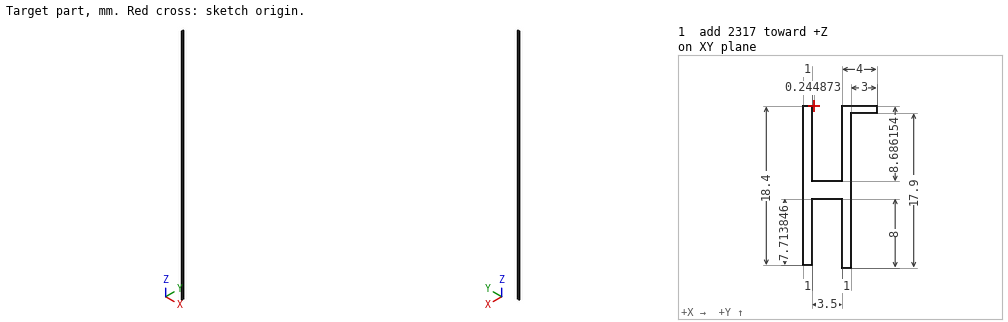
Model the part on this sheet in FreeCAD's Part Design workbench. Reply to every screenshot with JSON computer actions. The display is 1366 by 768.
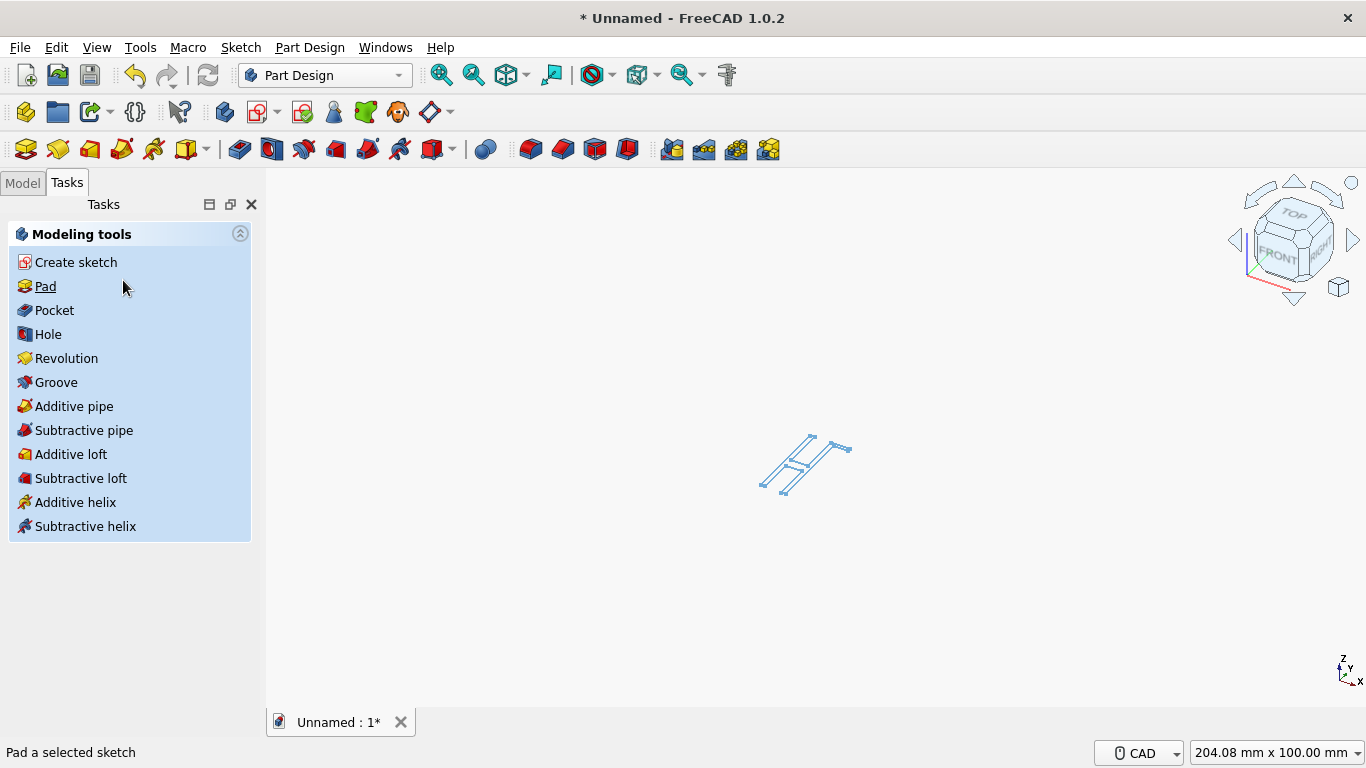
{"action": "left_click", "coordinate": [26, 150]}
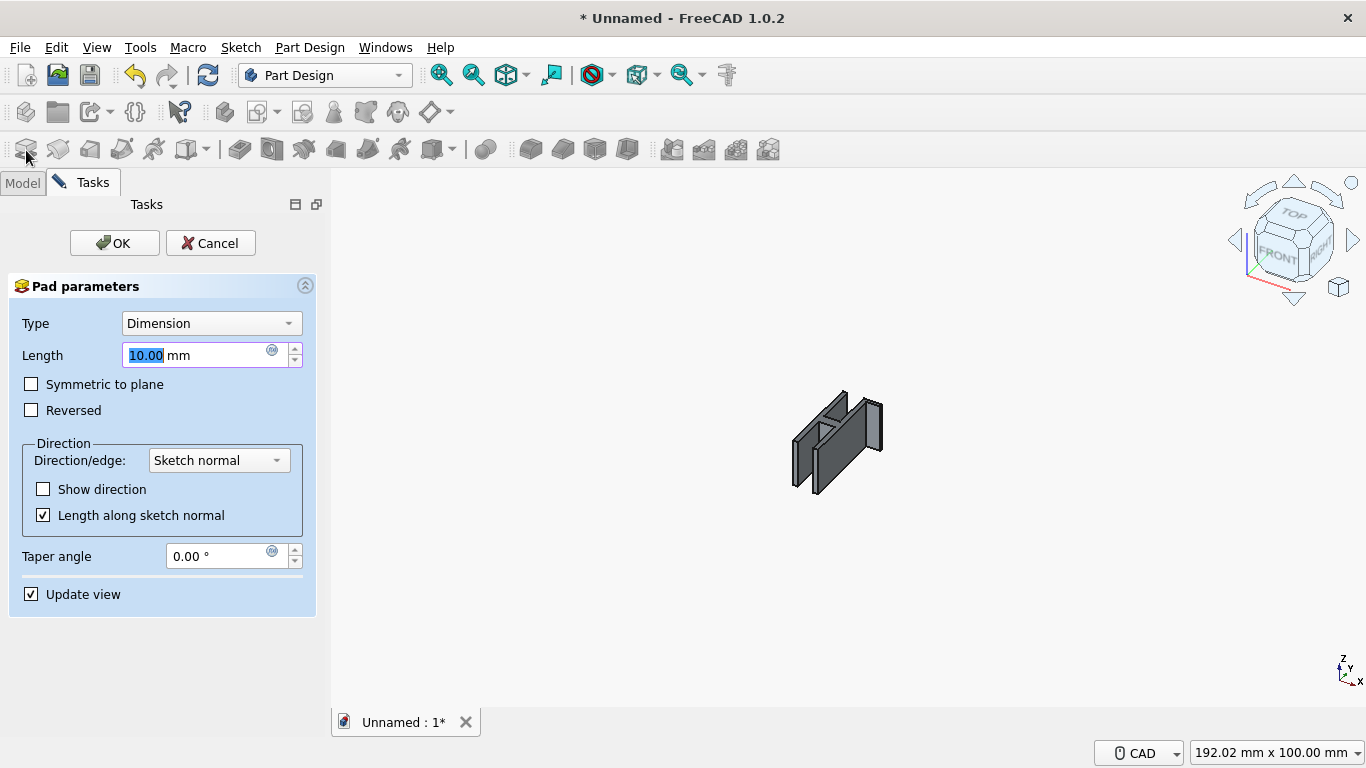
{"action": "type", "text": "2317"}
{"action": "key", "text": "Tab"}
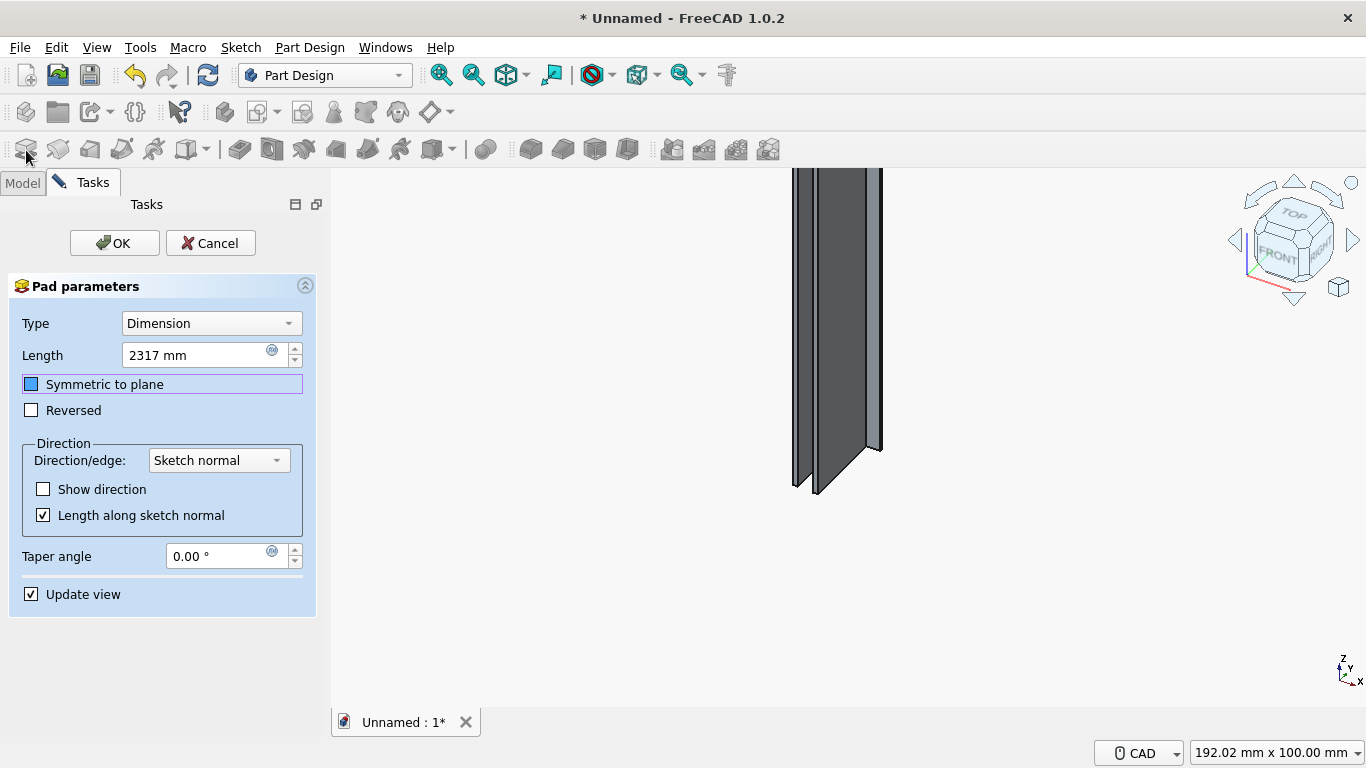
{"action": "left_click", "coordinate": [115, 243]}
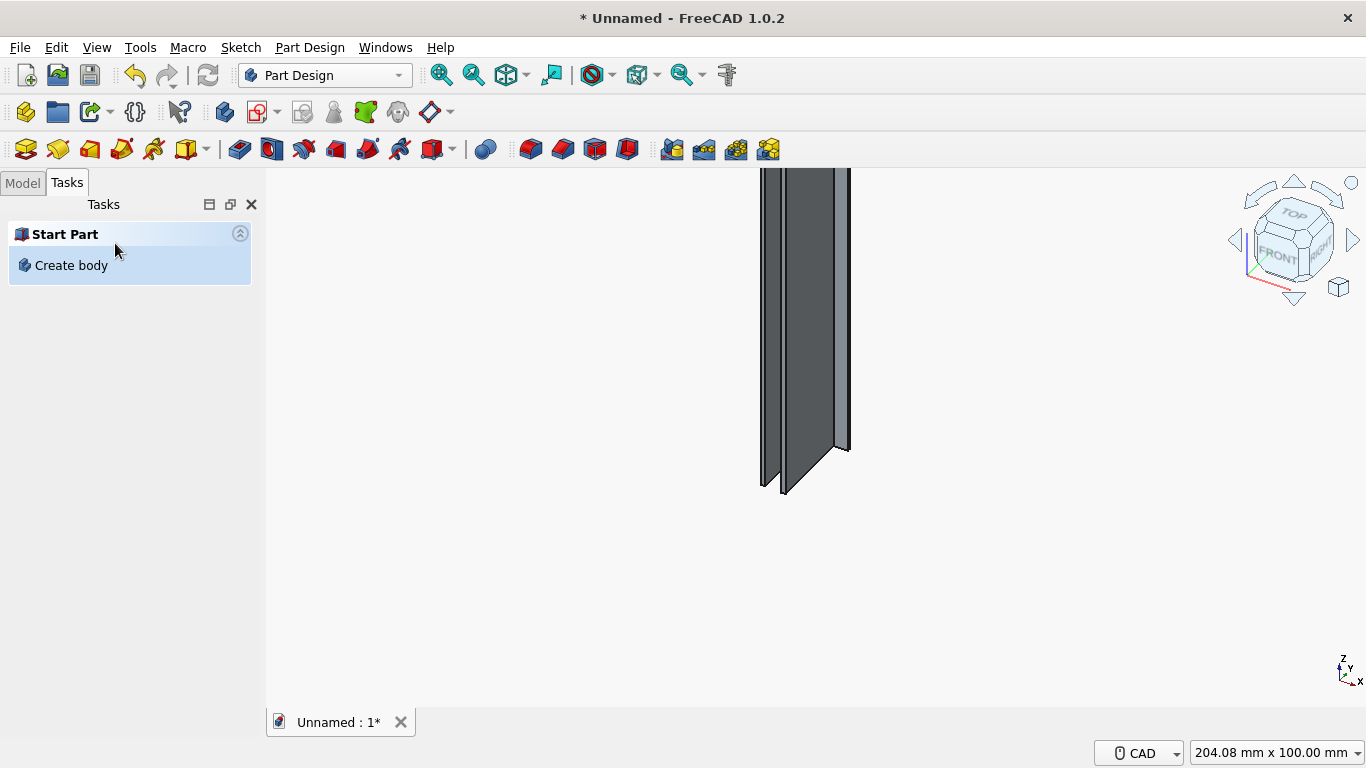
{"action": "key", "text": "0"}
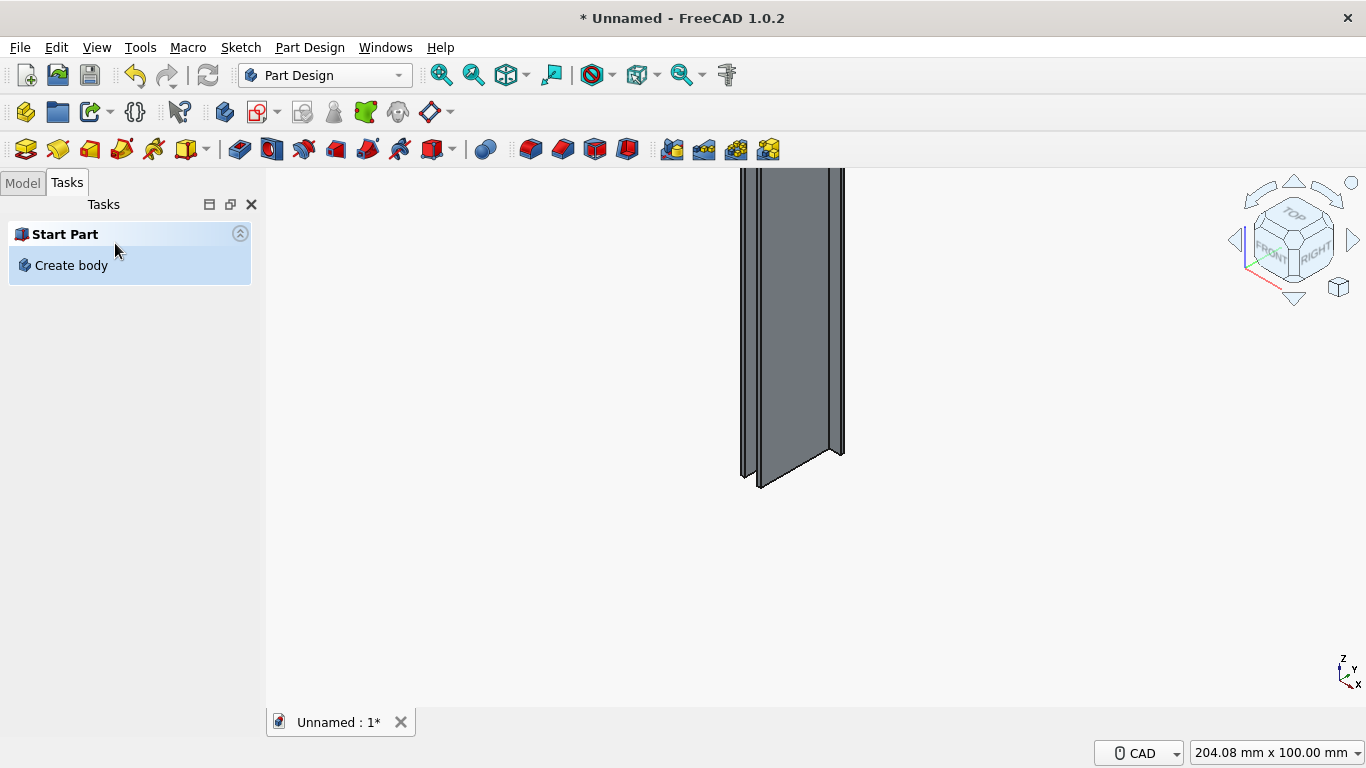
{"action": "key", "text": "v f"}